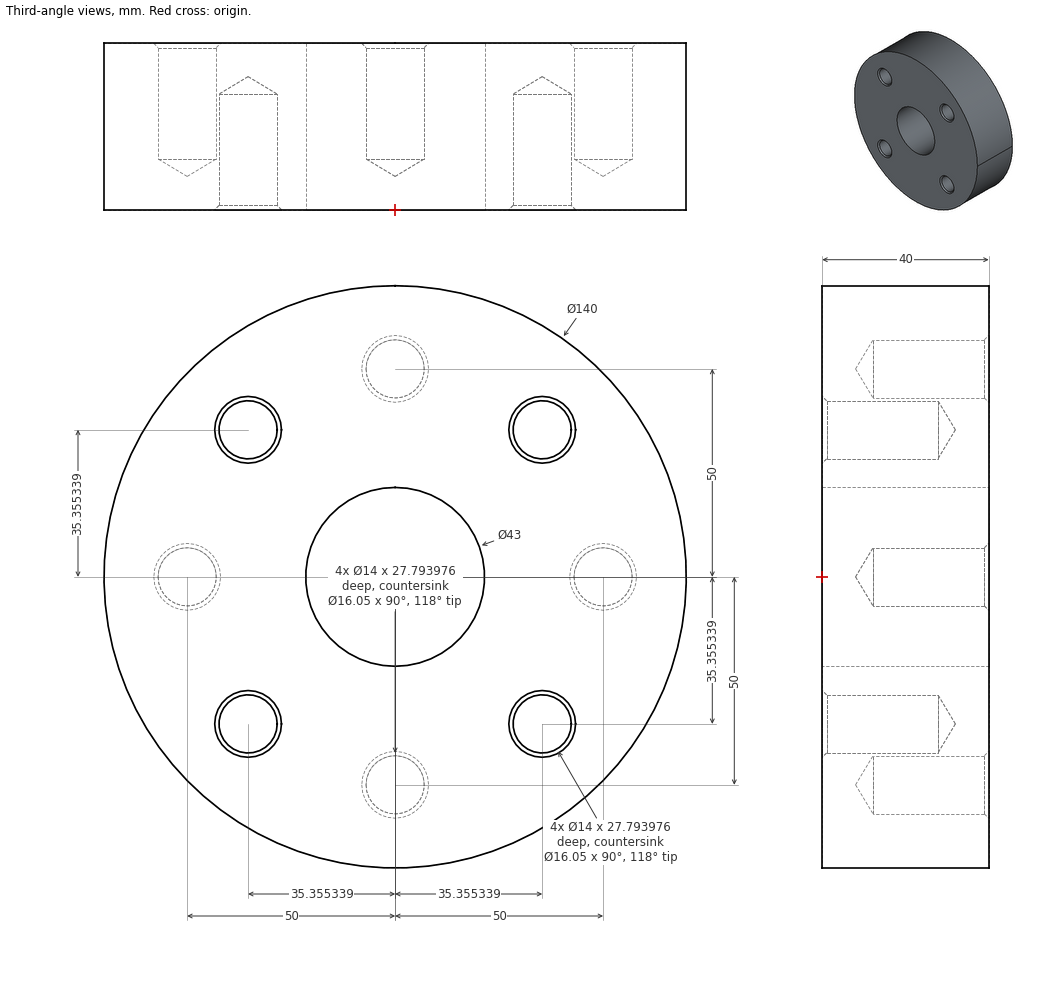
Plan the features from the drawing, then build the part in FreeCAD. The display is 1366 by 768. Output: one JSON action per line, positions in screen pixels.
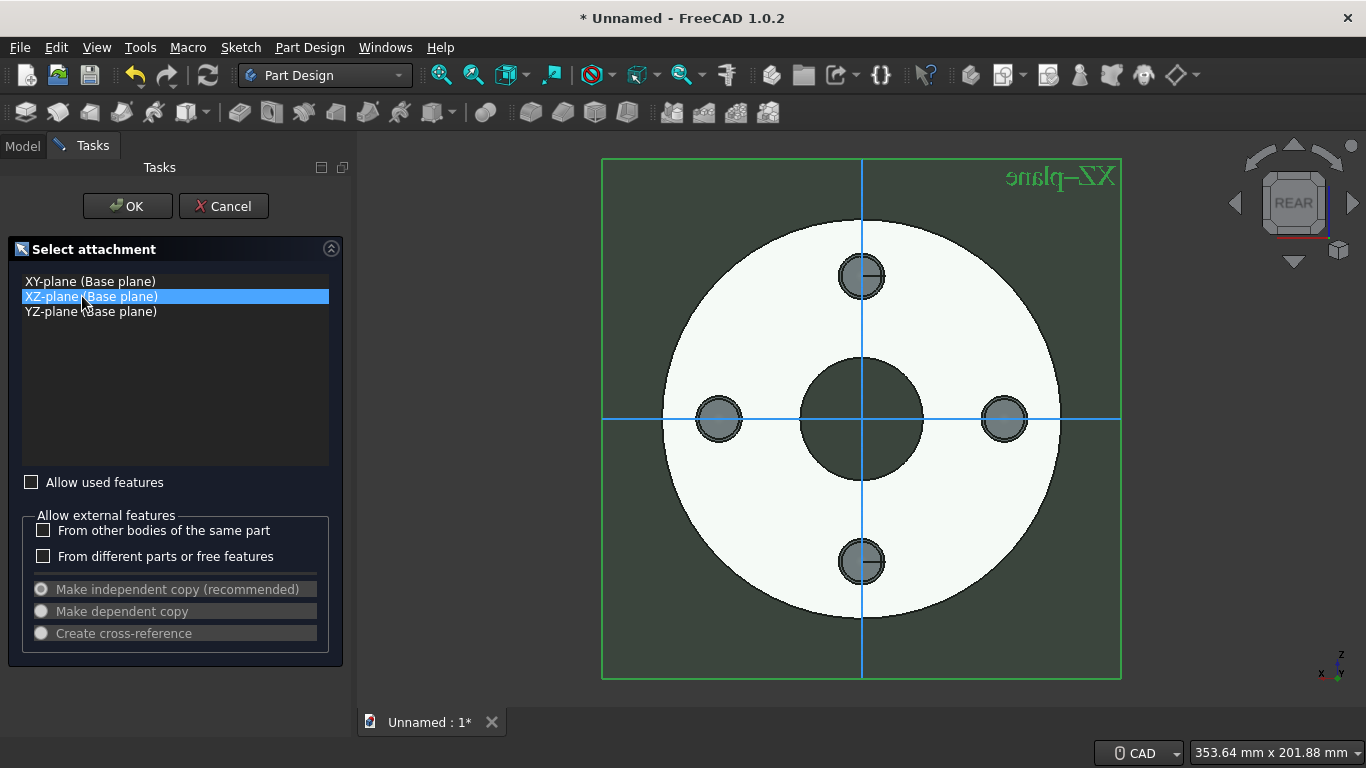
{"action": "left_click", "coordinate": [128, 206]}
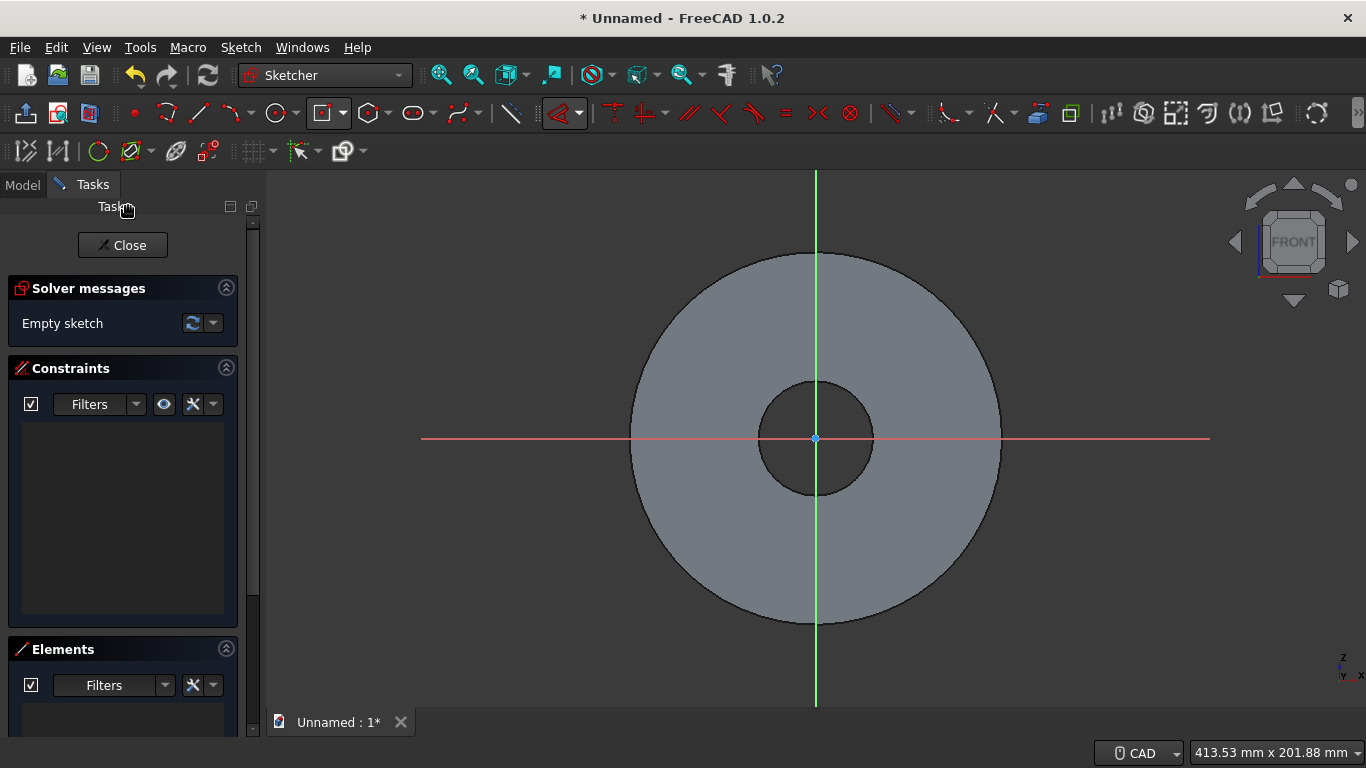
{"action": "scroll", "coordinate": [955, 439], "scroll_direction": "up", "scroll_amount": 2}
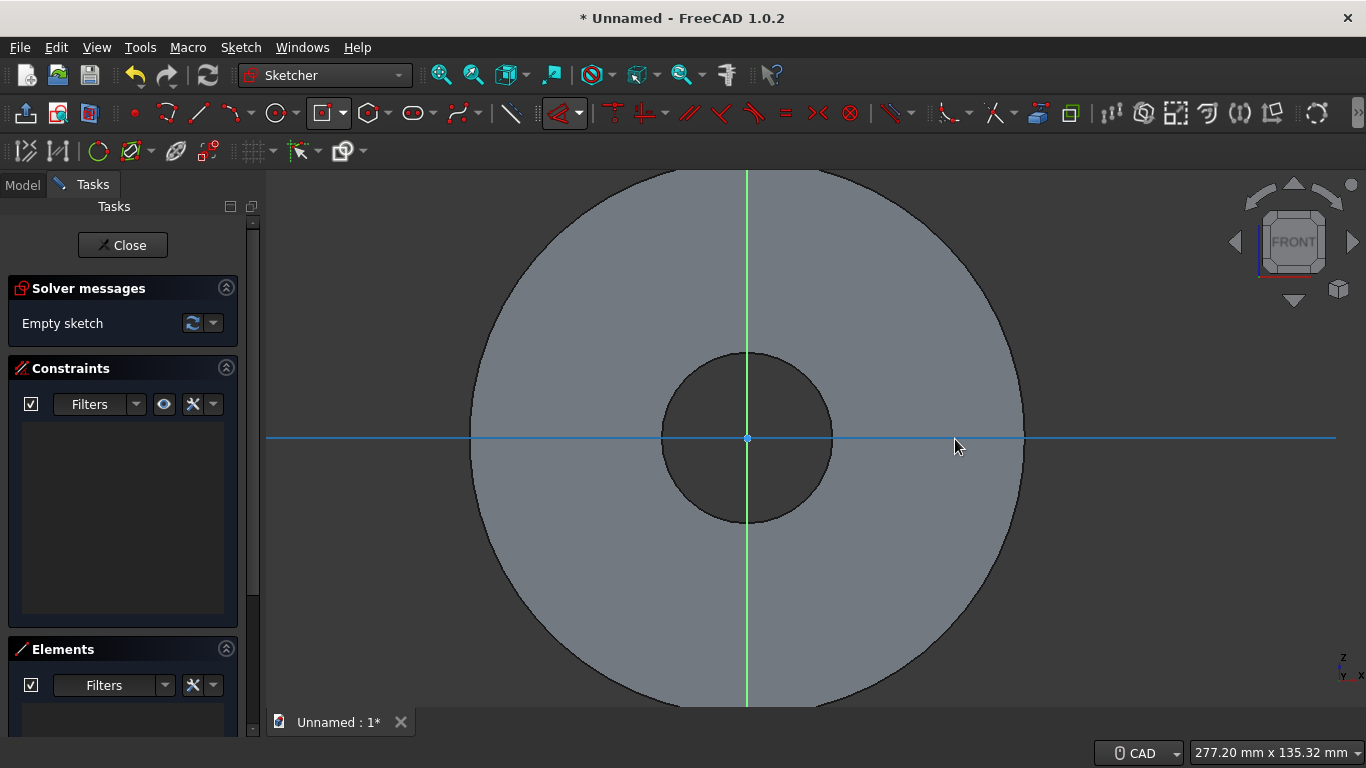
{"action": "left_click", "coordinate": [276, 114]}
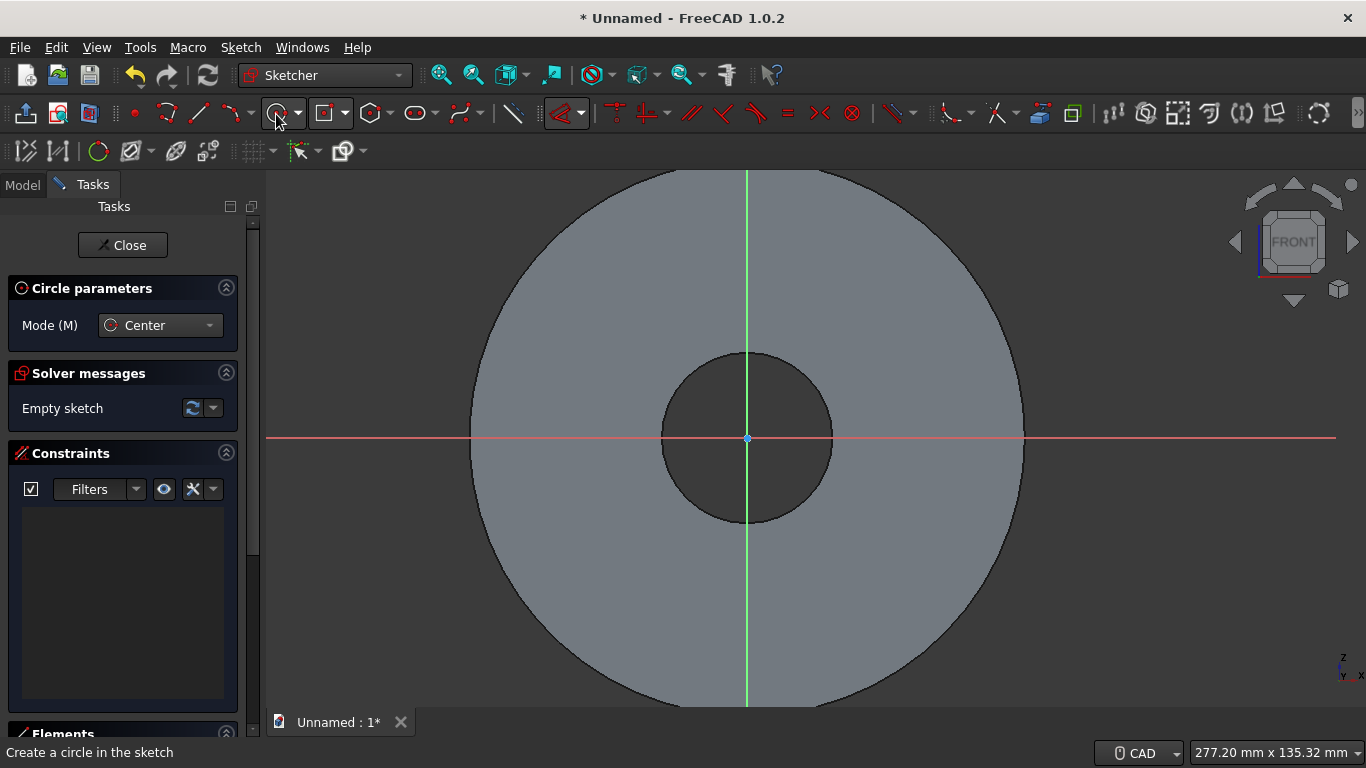
{"action": "left_click", "coordinate": [887, 578]}
{"action": "mouse_move", "coordinate": [907, 559]}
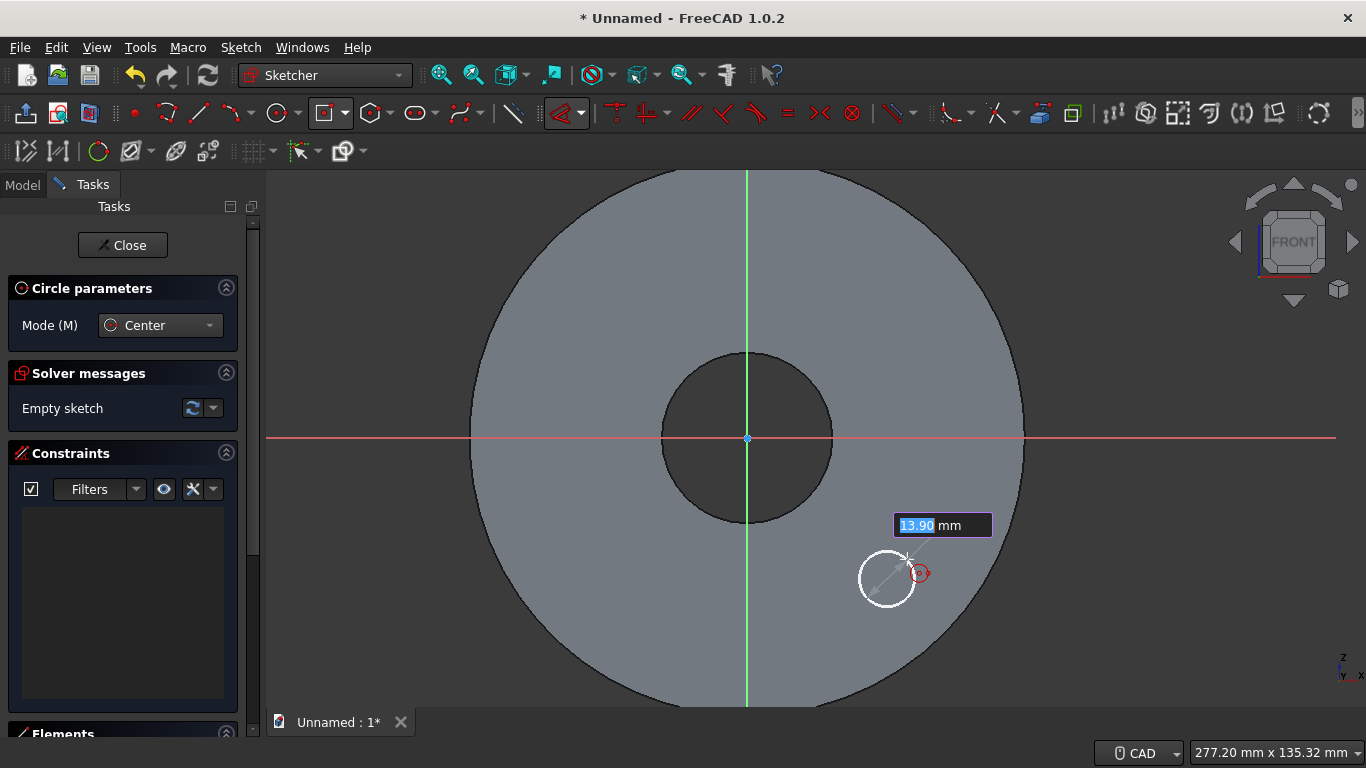
{"action": "type", "text": "14"}
{"action": "key", "text": "Return"}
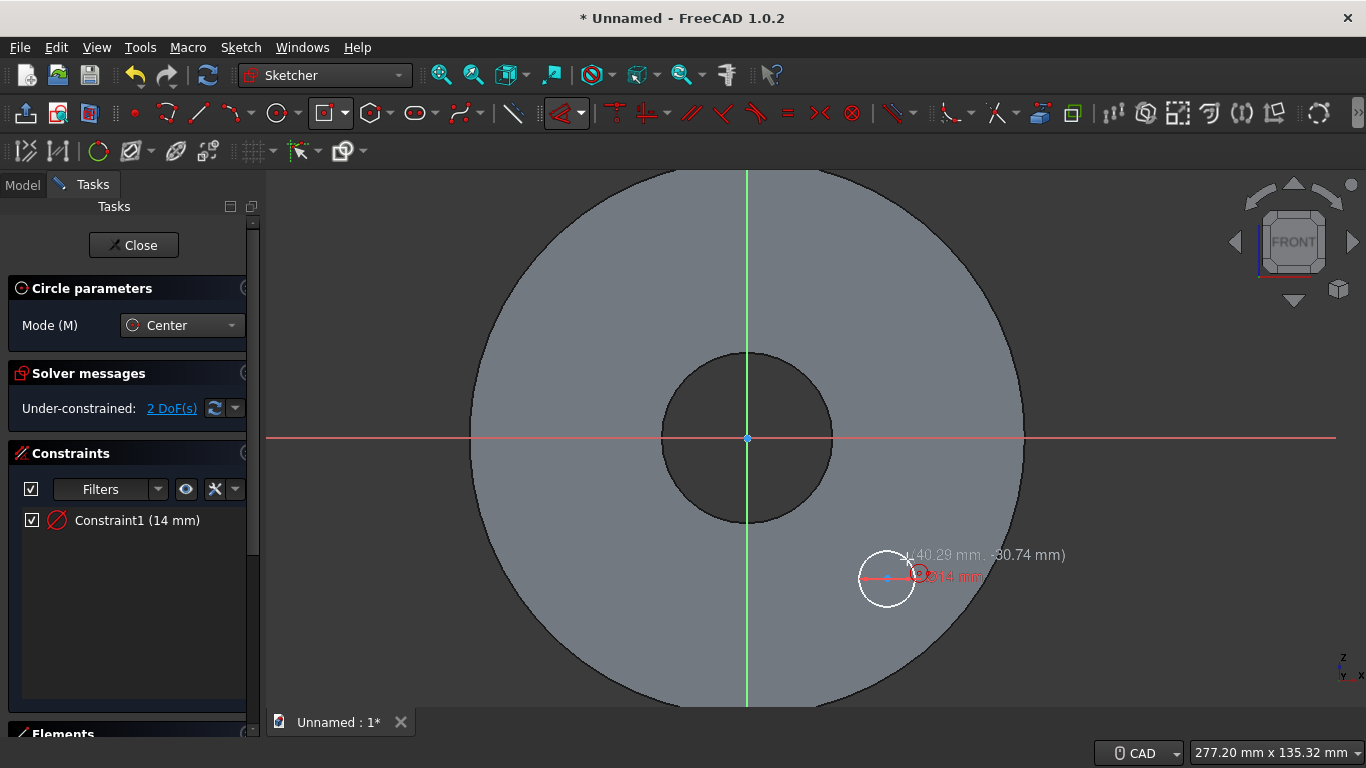
{"action": "left_click", "coordinate": [607, 578]}
{"action": "mouse_move", "coordinate": [626, 559]}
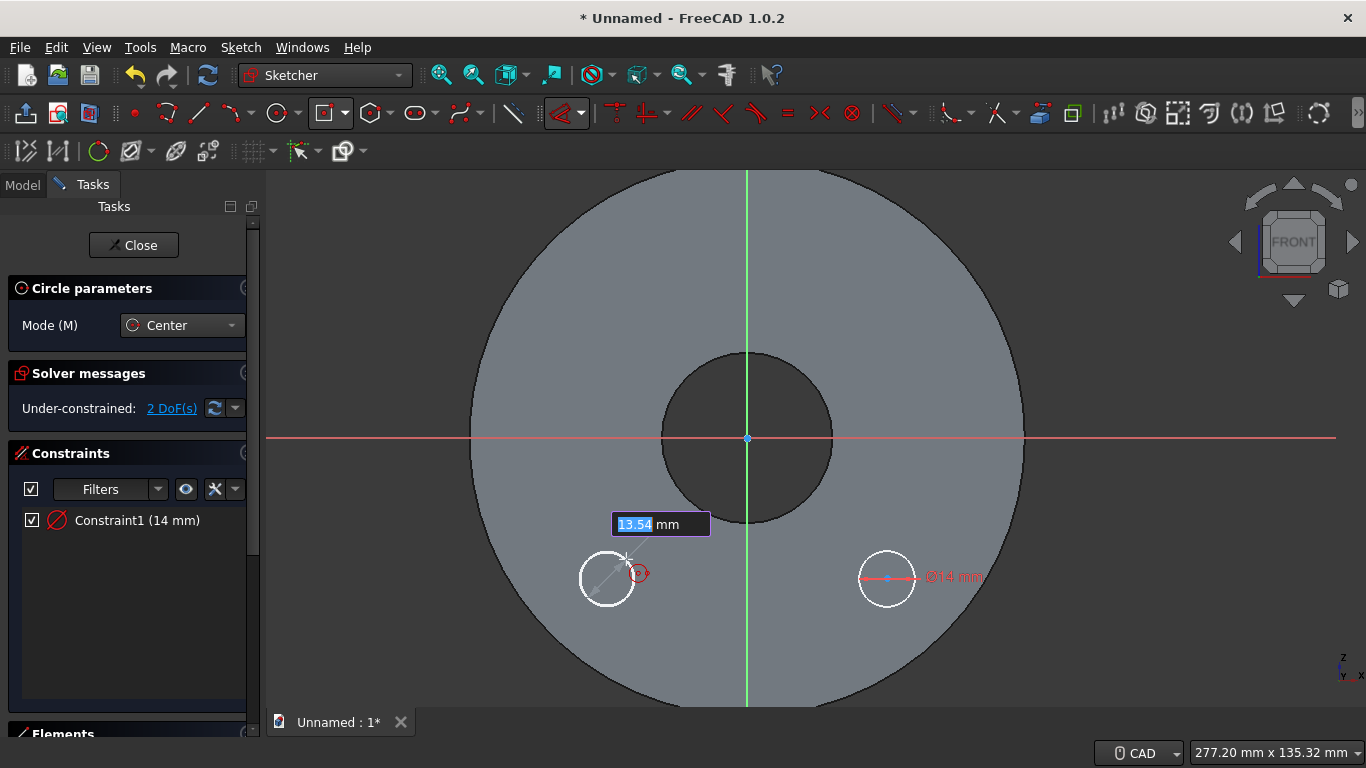
{"action": "type", "text": "14"}
{"action": "key", "text": "Return"}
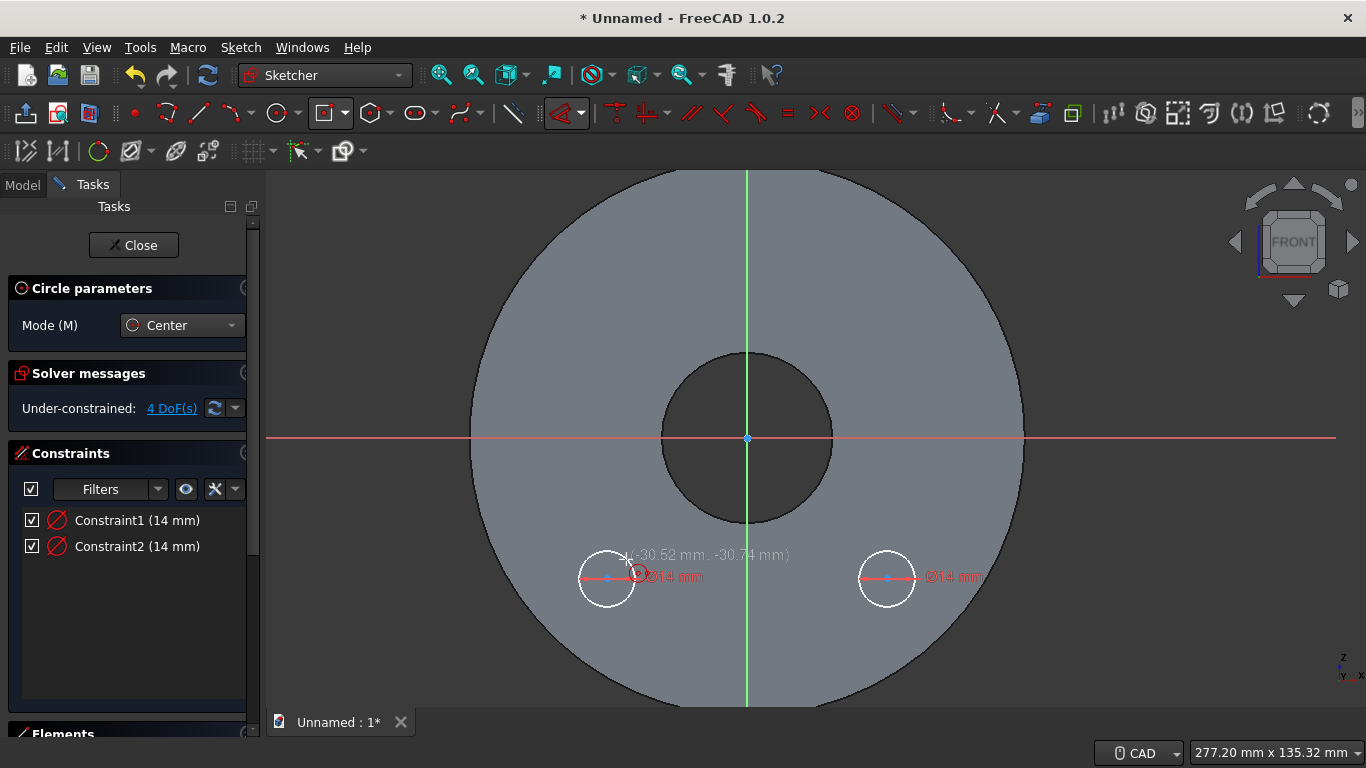
{"action": "left_click", "coordinate": [607, 298]}
{"action": "mouse_move", "coordinate": [626, 278]}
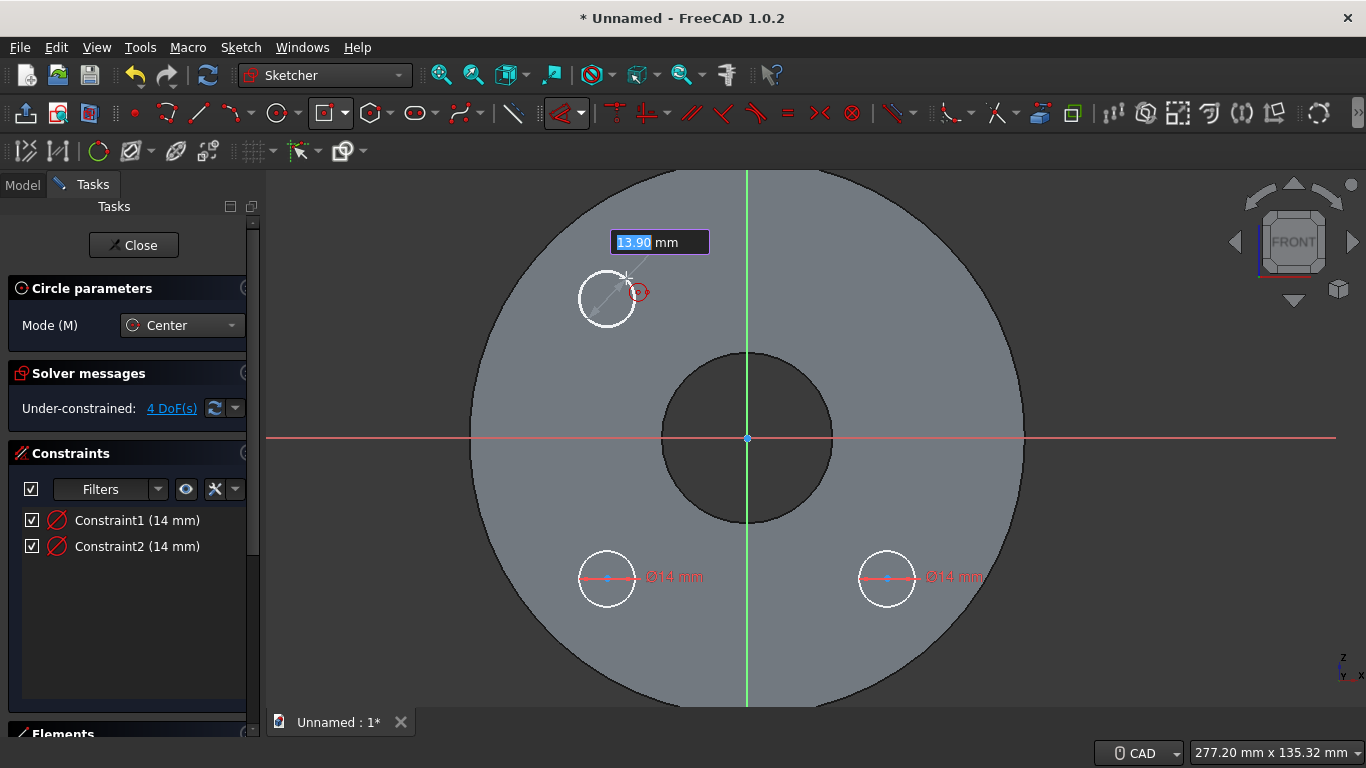
{"action": "type", "text": "14"}
{"action": "key", "text": "Return"}